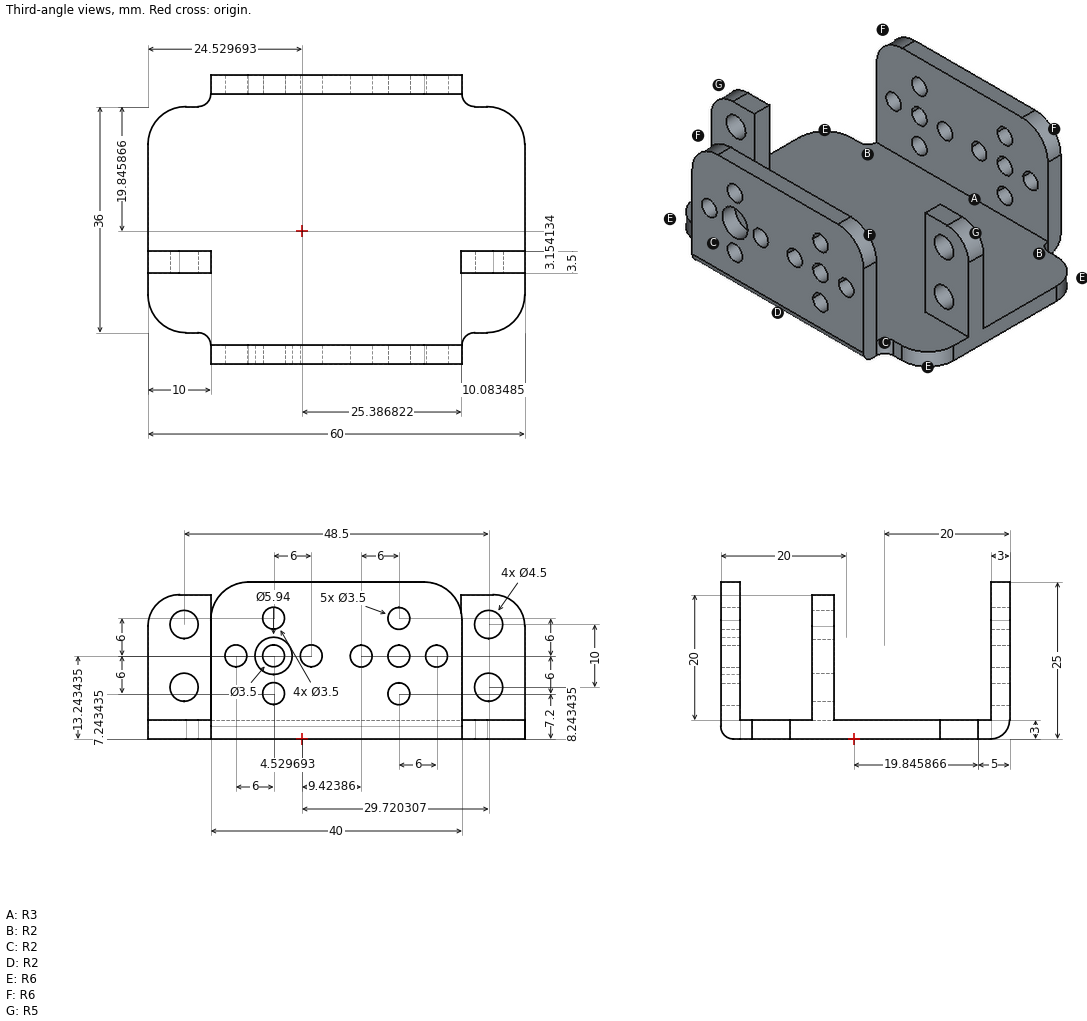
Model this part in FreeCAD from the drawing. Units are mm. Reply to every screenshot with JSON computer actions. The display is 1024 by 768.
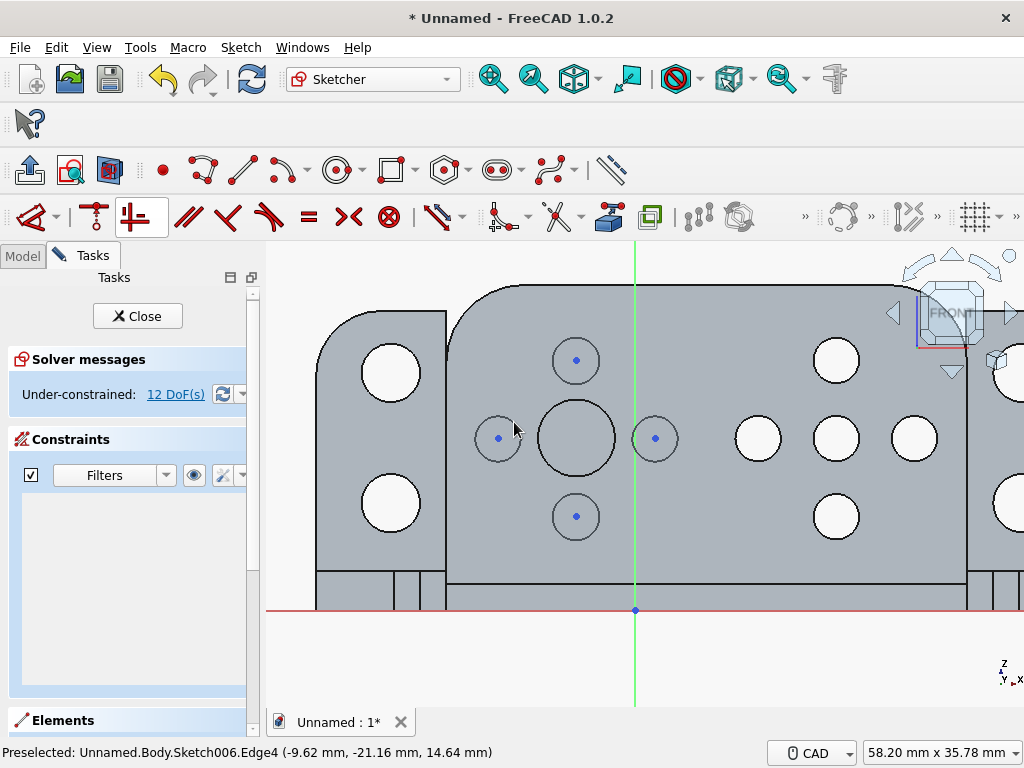
{"action": "left_click", "coordinate": [592, 344]}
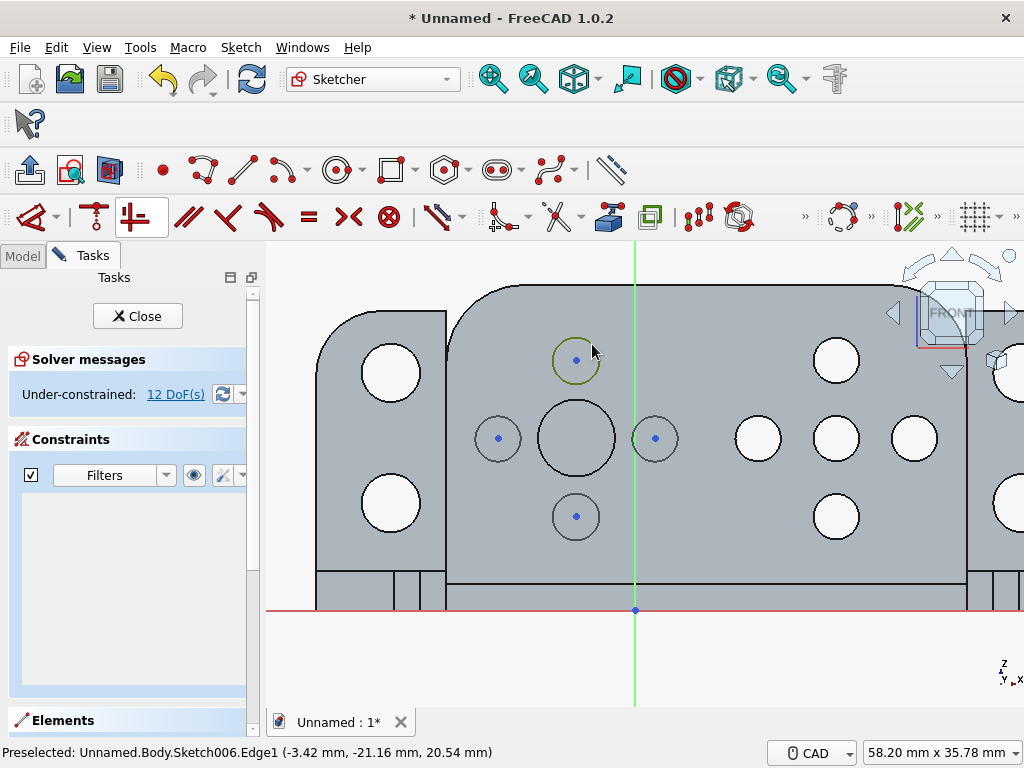
{"action": "left_click", "coordinate": [671, 423]}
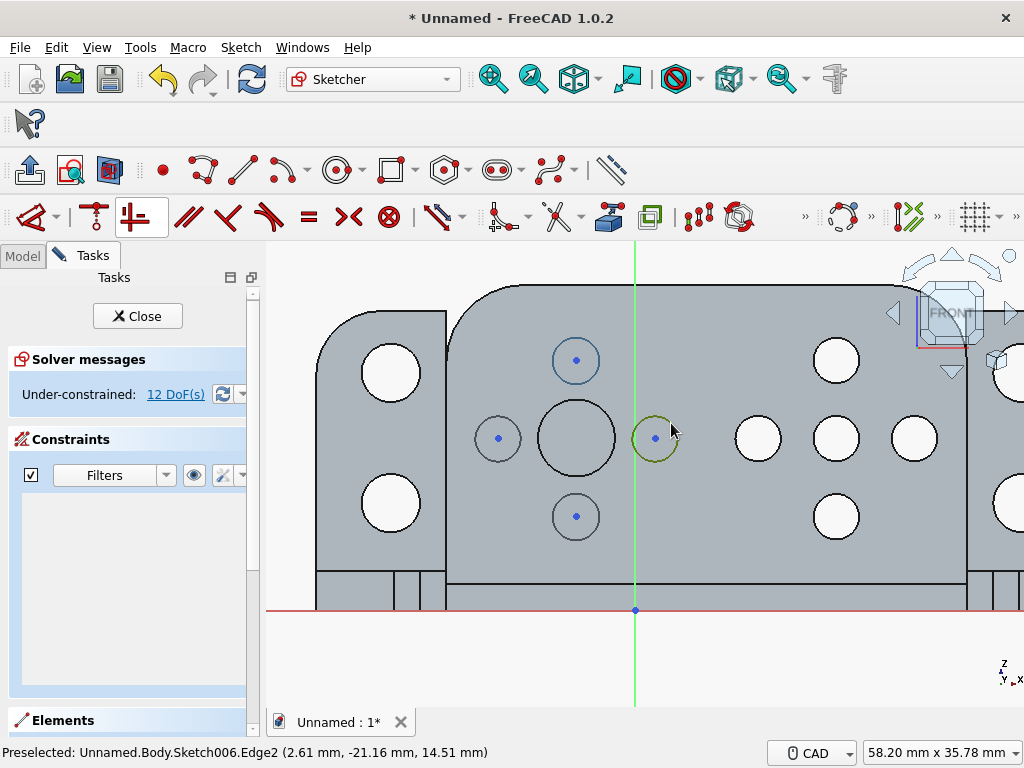
{"action": "left_click", "coordinate": [592, 500]}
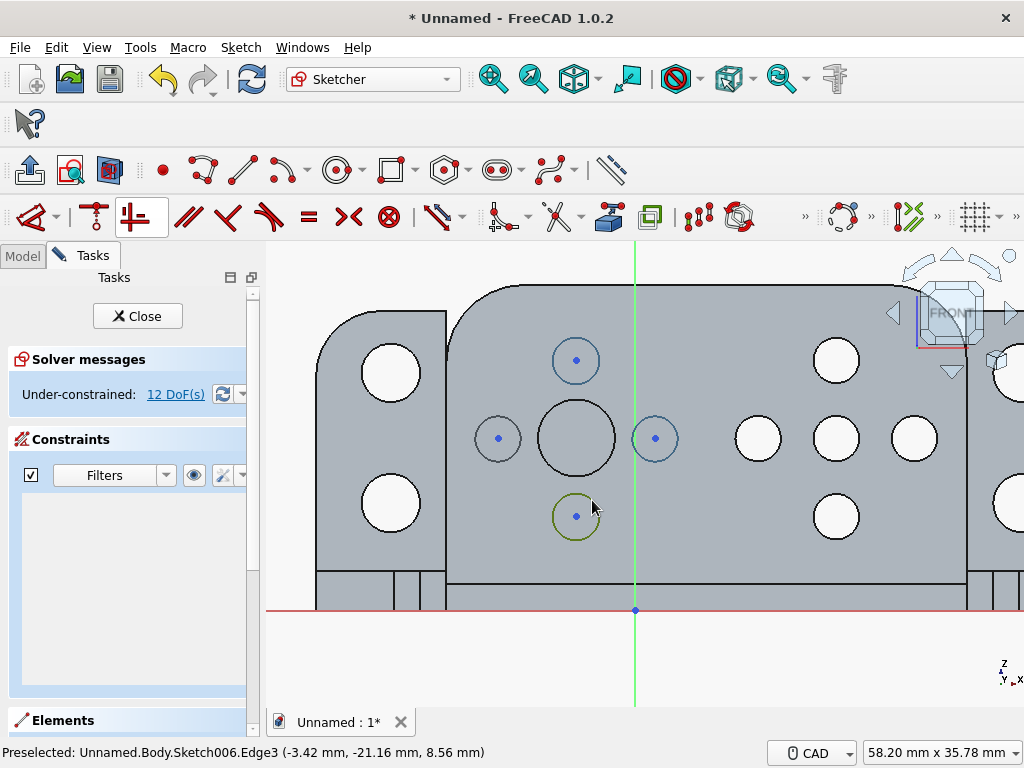
{"action": "left_click", "coordinate": [514, 423]}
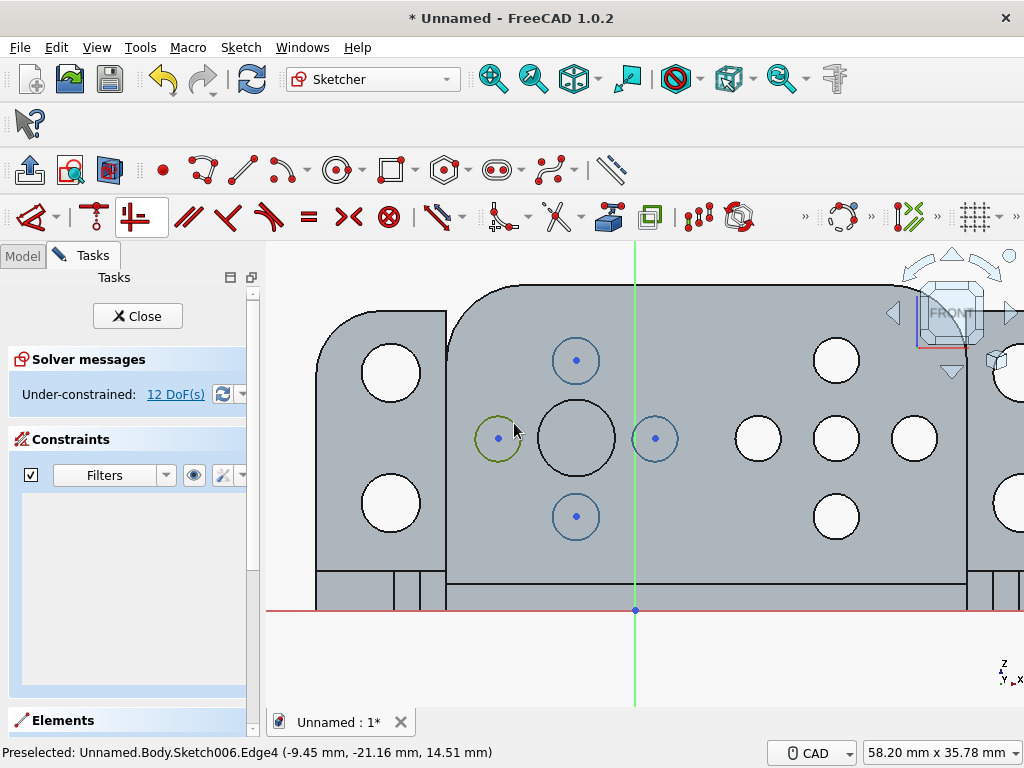
{"action": "left_click", "coordinate": [310, 218]}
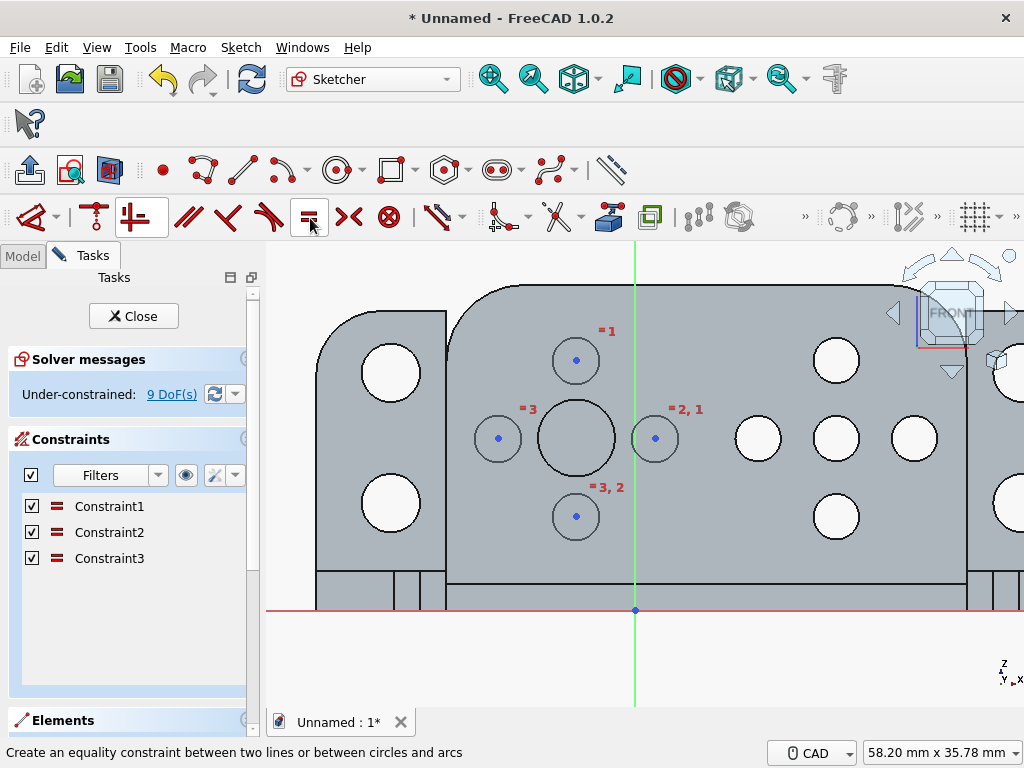
{"action": "left_click", "coordinate": [576, 361]}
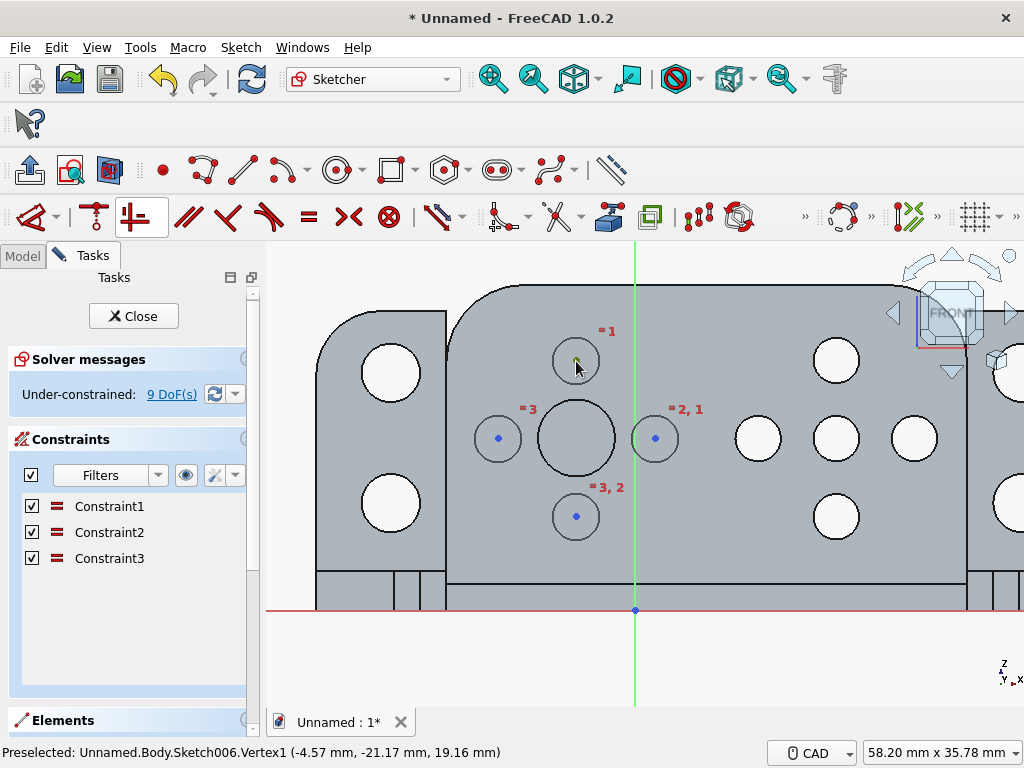
{"action": "left_click", "coordinate": [576, 517]}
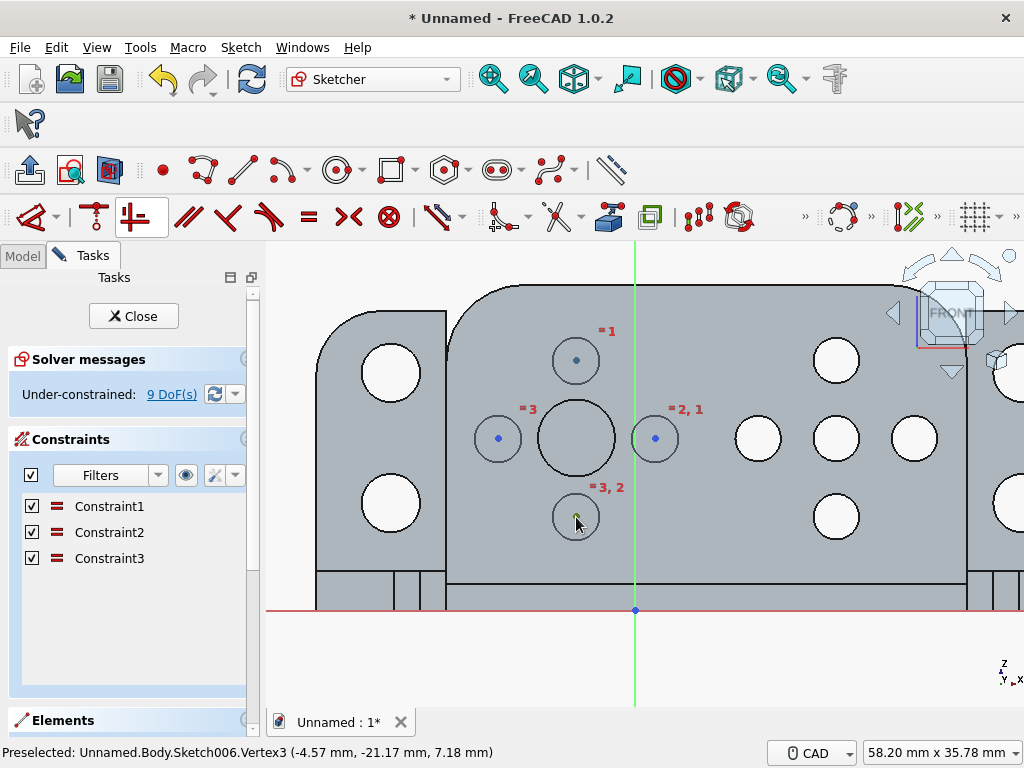
{"action": "key", "text": "v"}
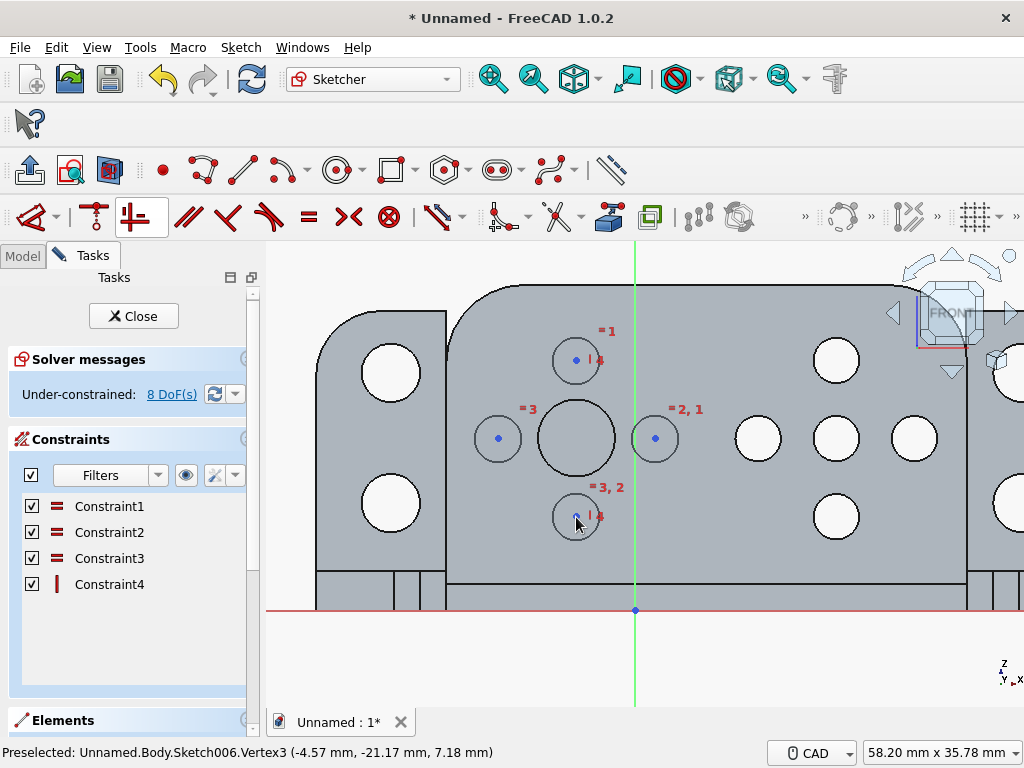
{"action": "left_click", "coordinate": [655, 439]}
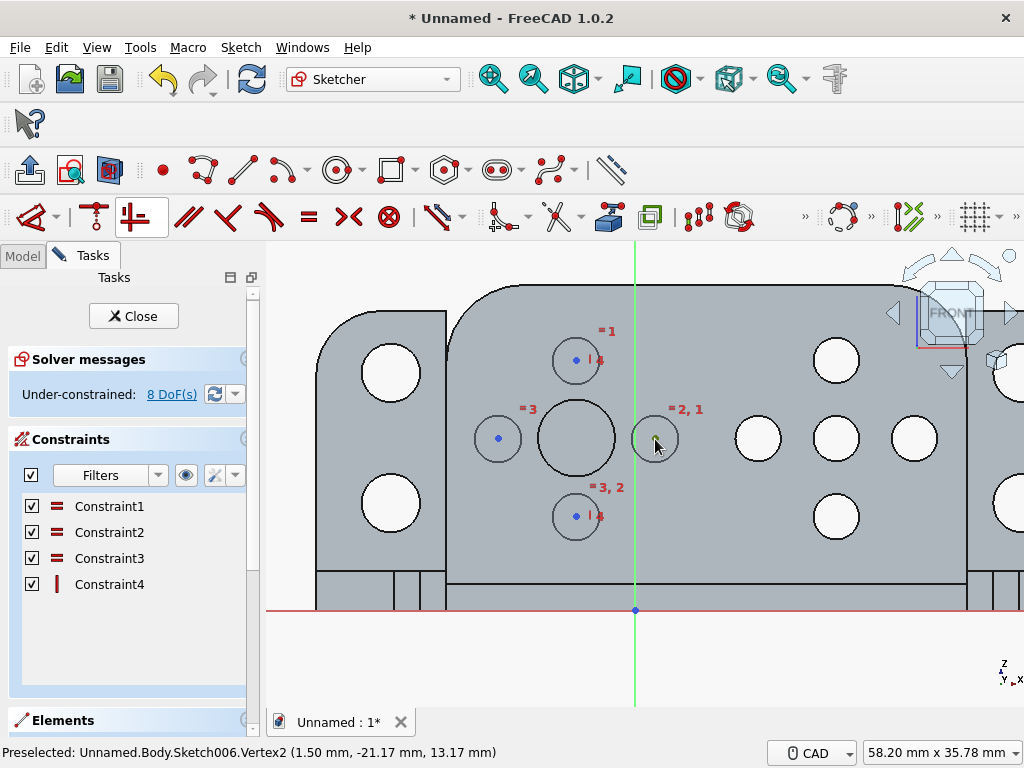
{"action": "left_click", "coordinate": [498, 439]}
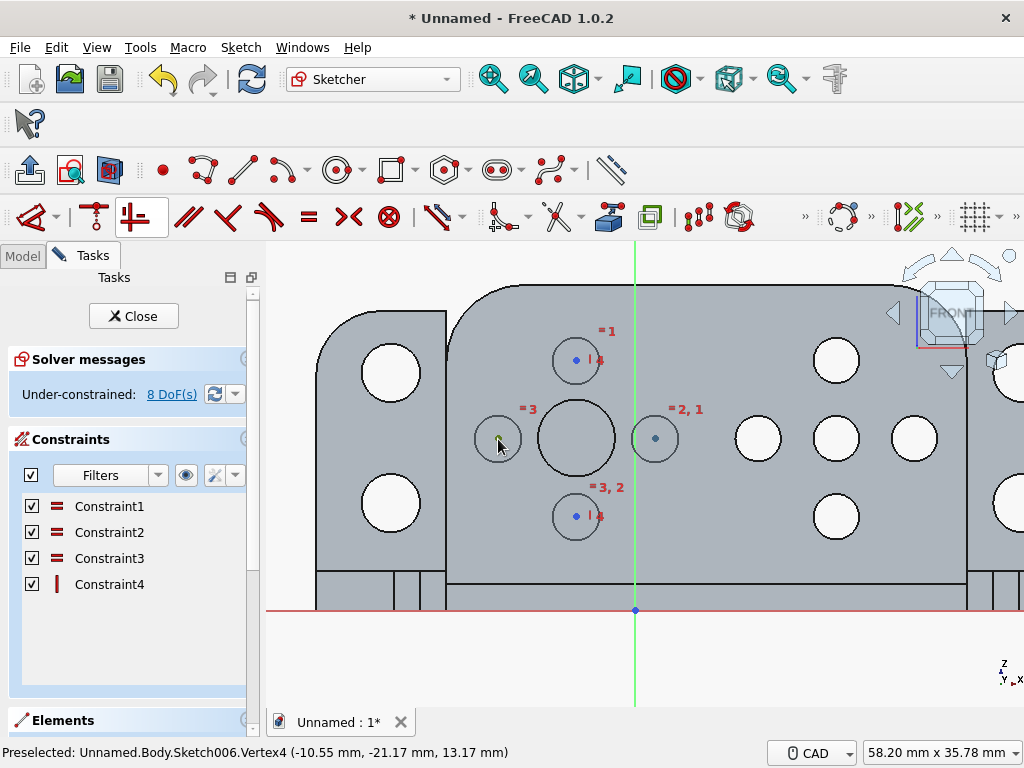
{"action": "left_click", "coordinate": [162, 218]}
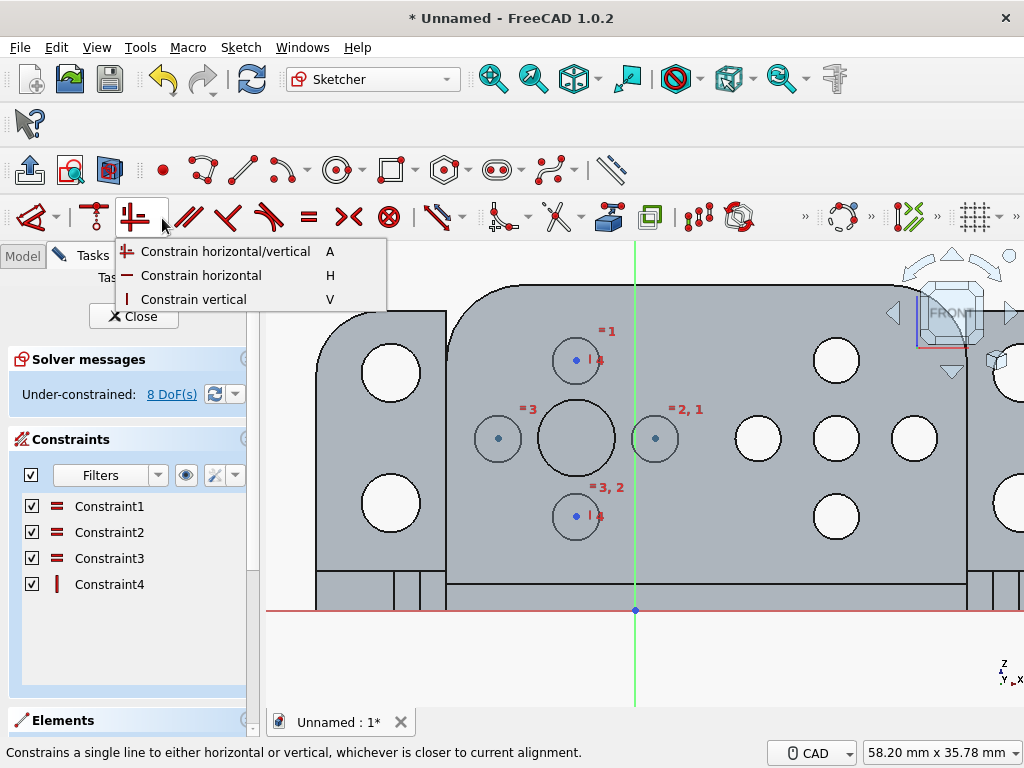
{"action": "left_click", "coordinate": [251, 275]}